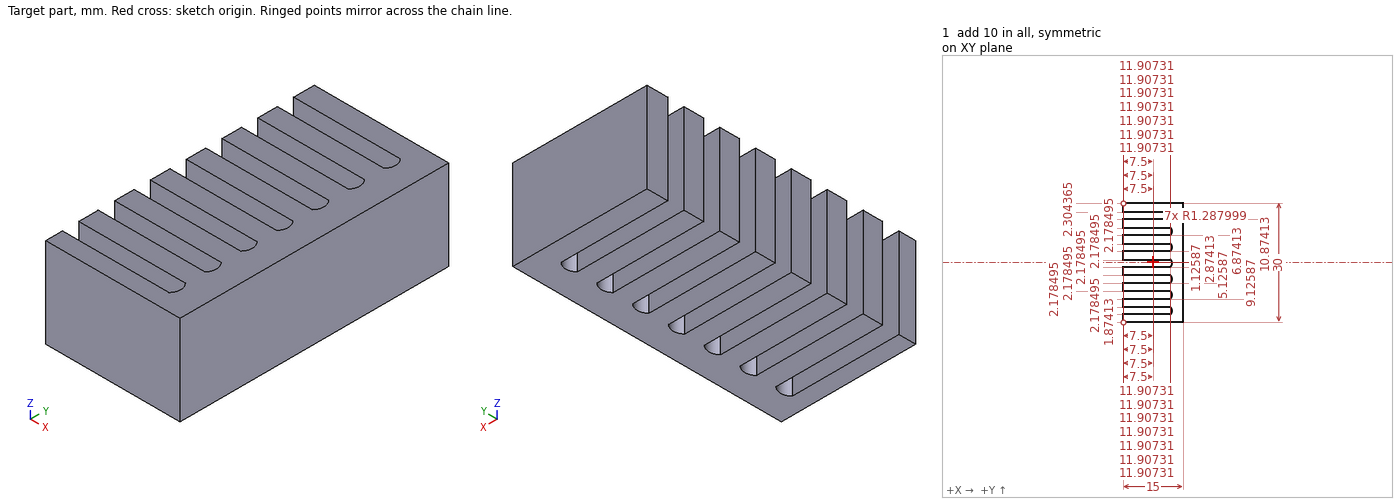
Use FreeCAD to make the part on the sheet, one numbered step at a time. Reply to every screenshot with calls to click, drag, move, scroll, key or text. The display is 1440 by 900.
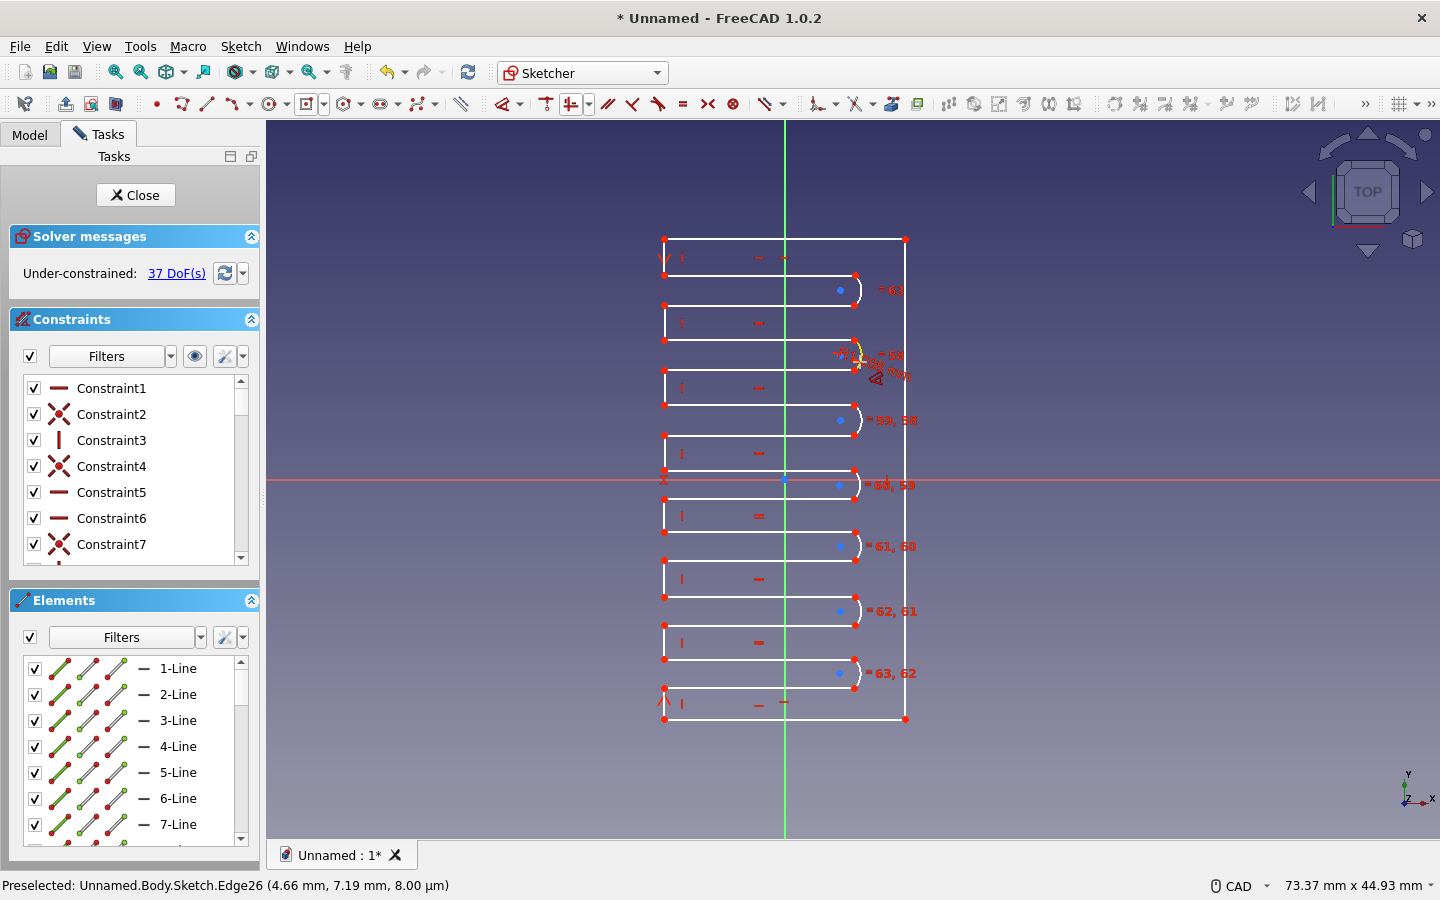
click(737, 720)
click(729, 754)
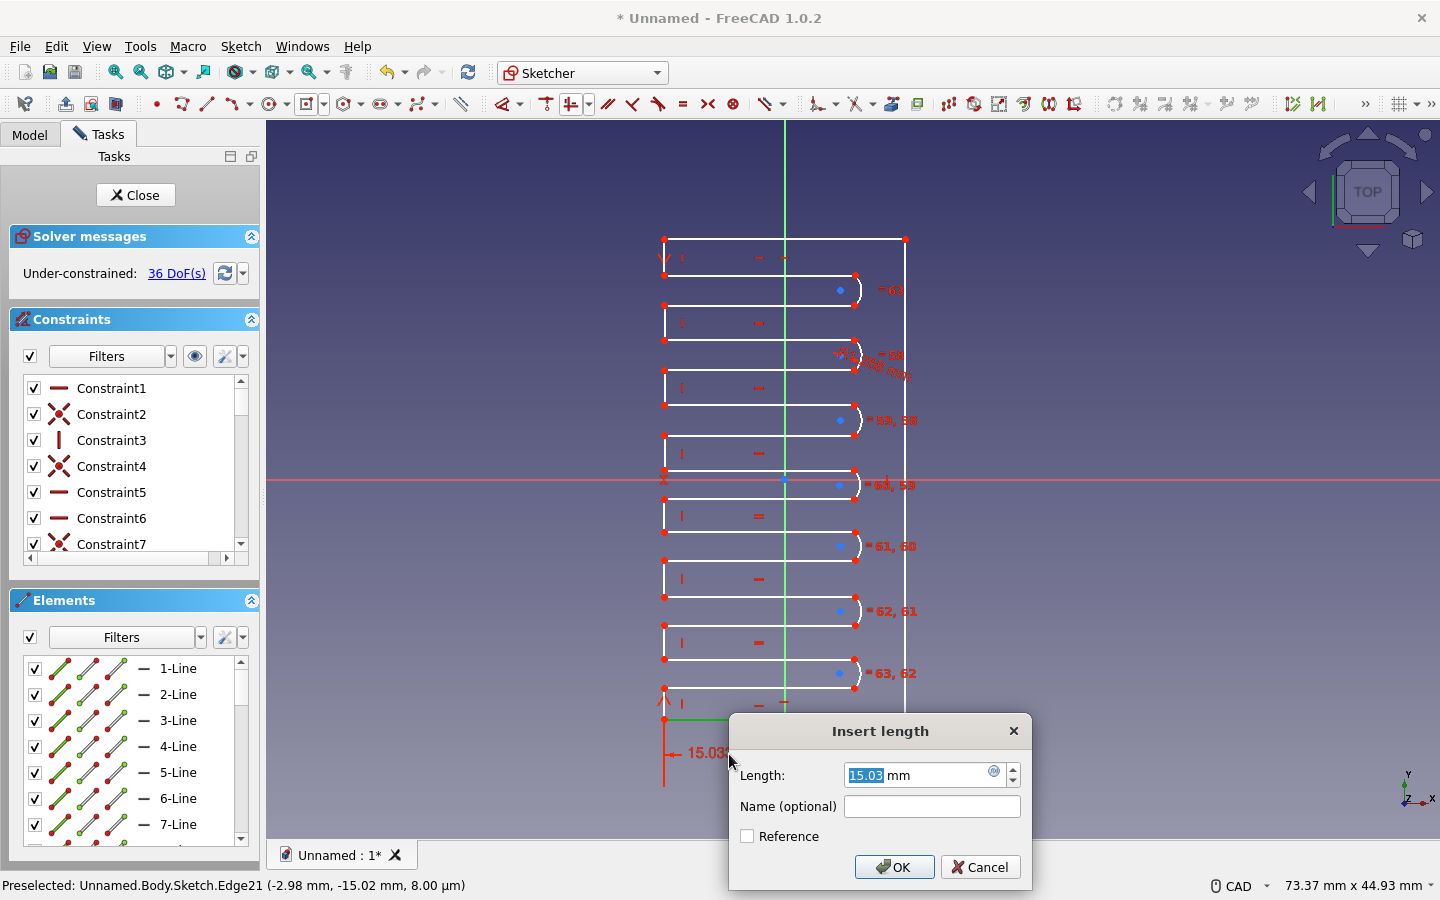
text(15)
key(Return)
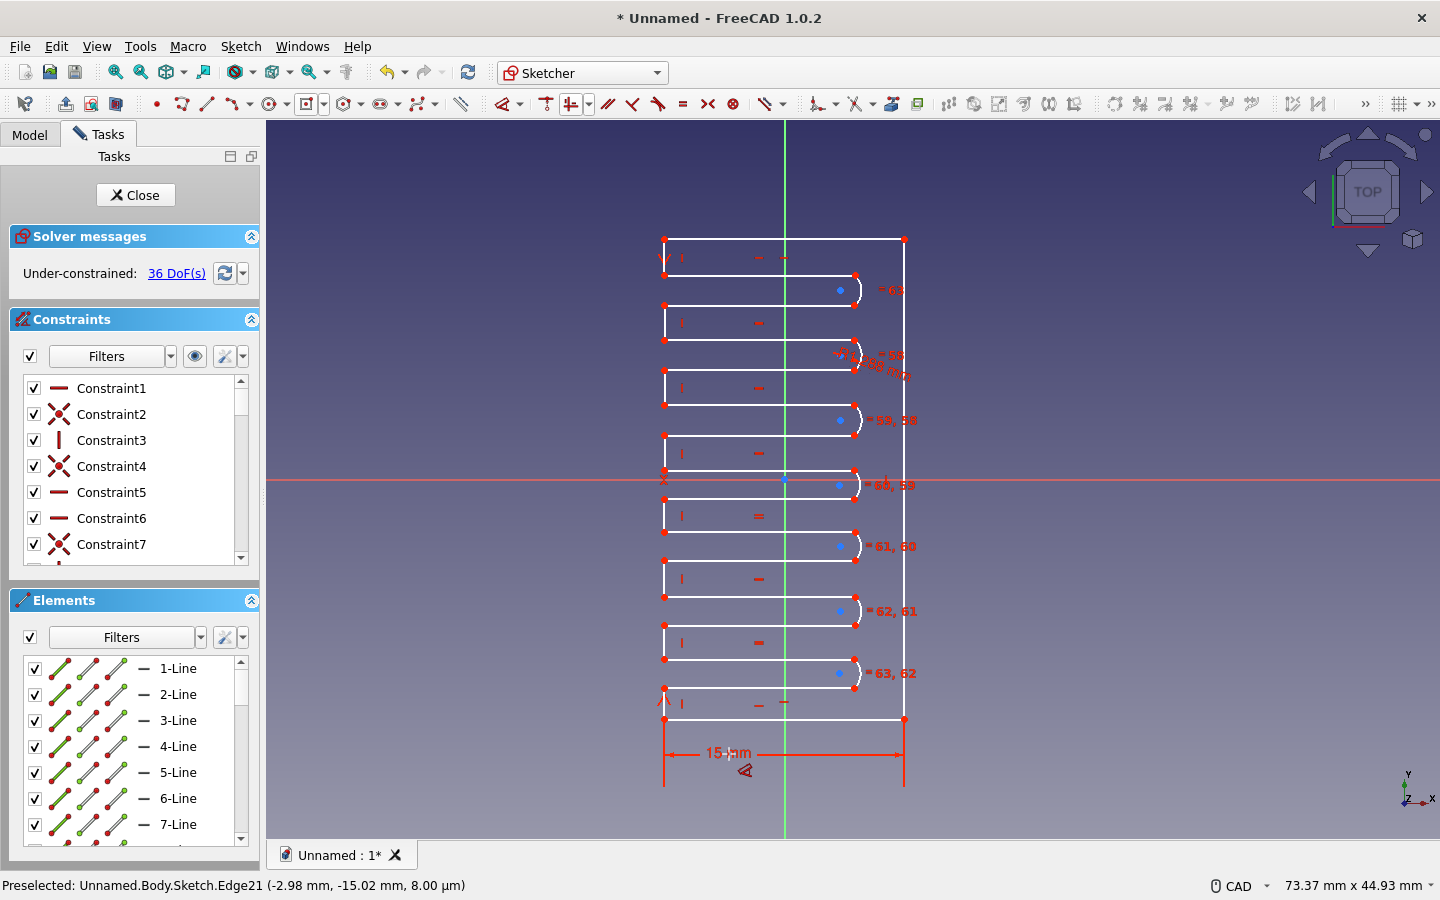
click(904, 576)
click(938, 590)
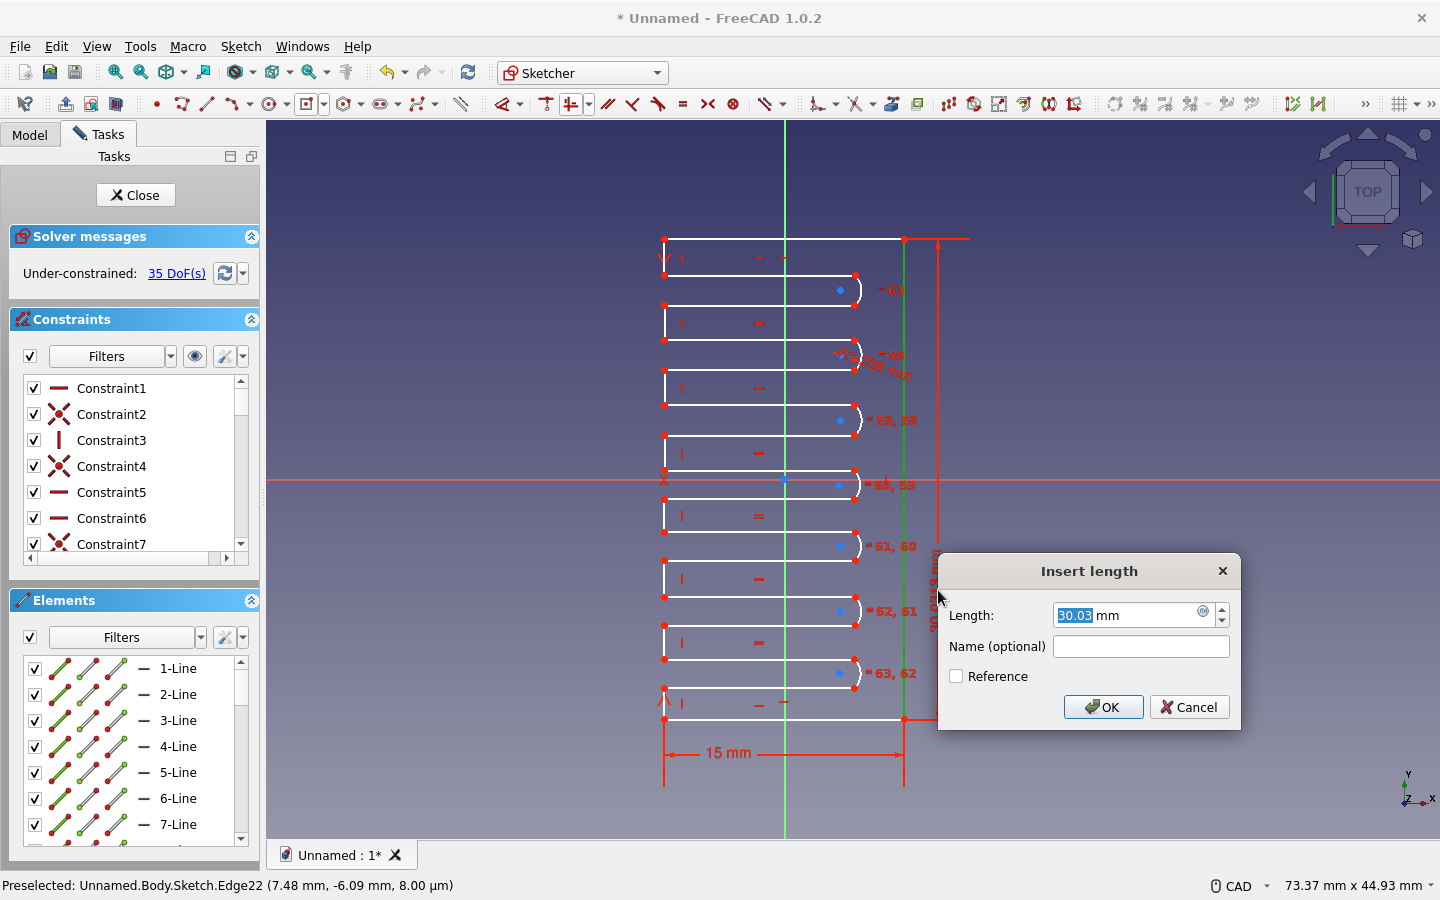
text(30)
key(Return)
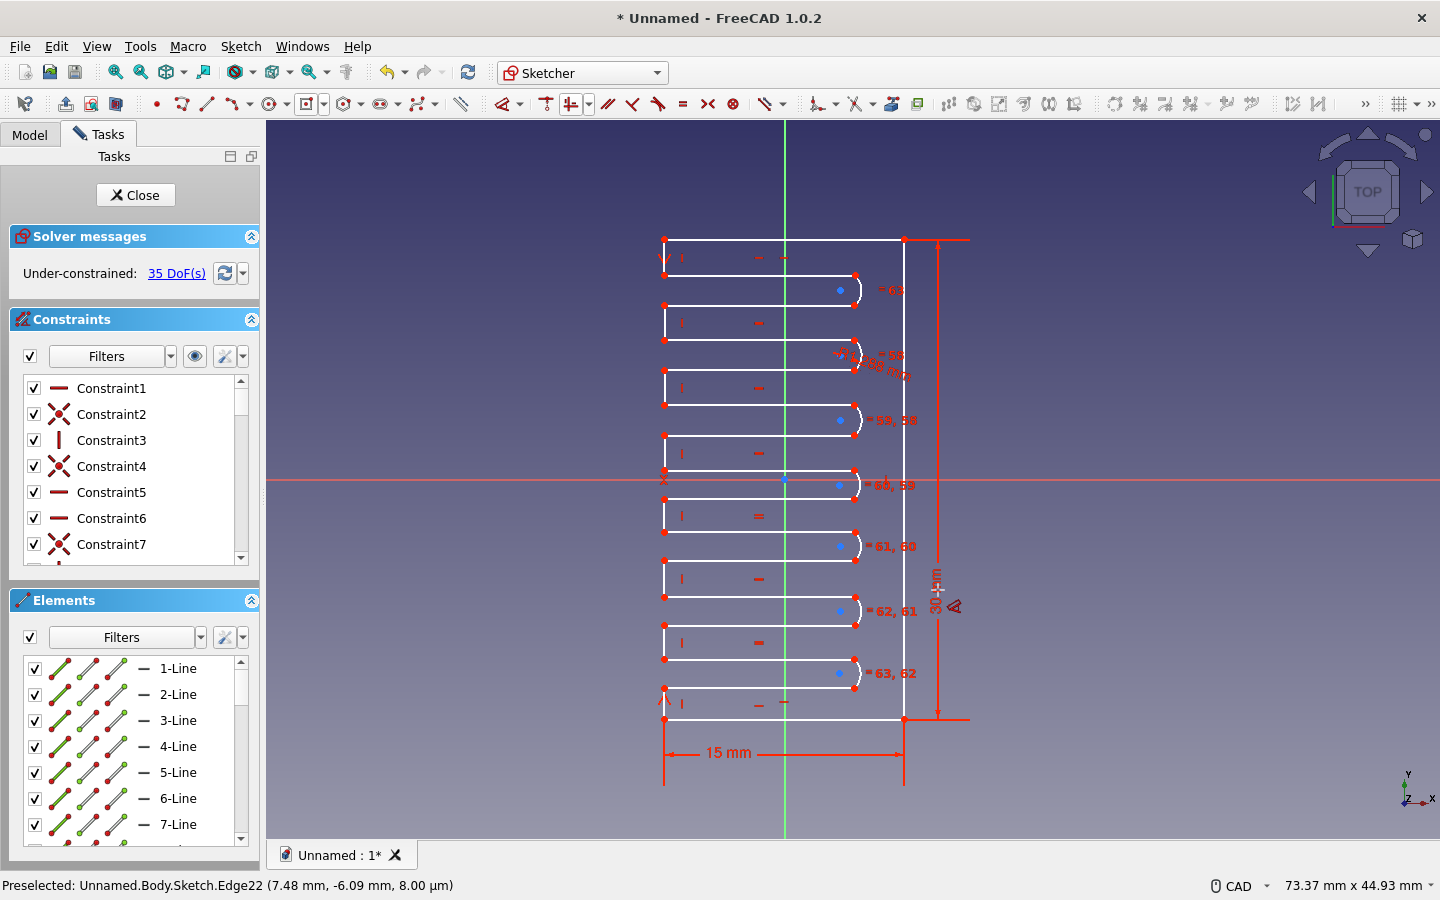
click(665, 306)
click(725, 514)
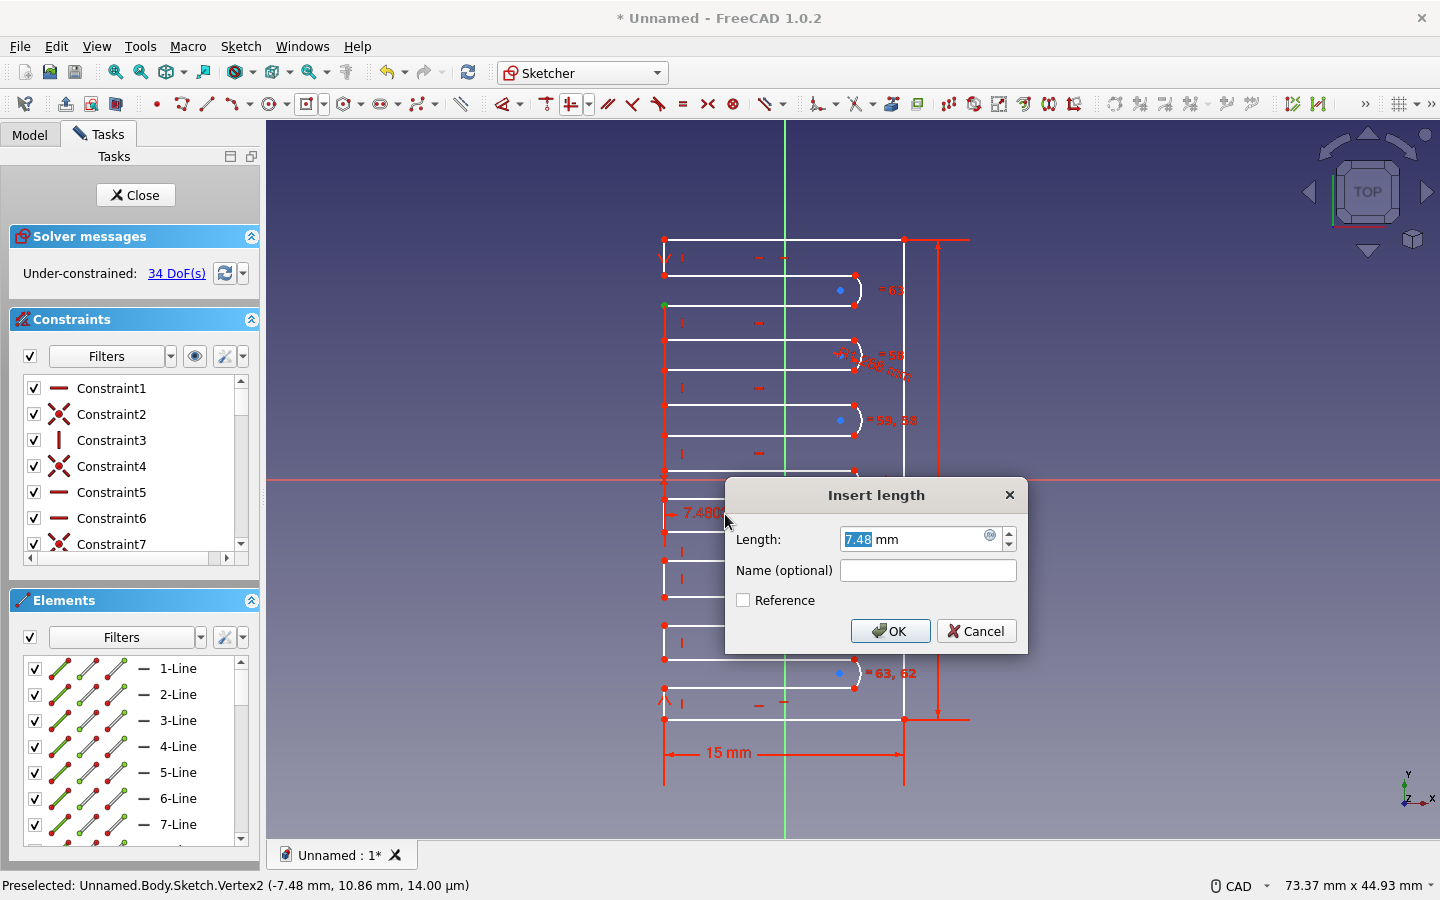
text(7.5)
key(Return)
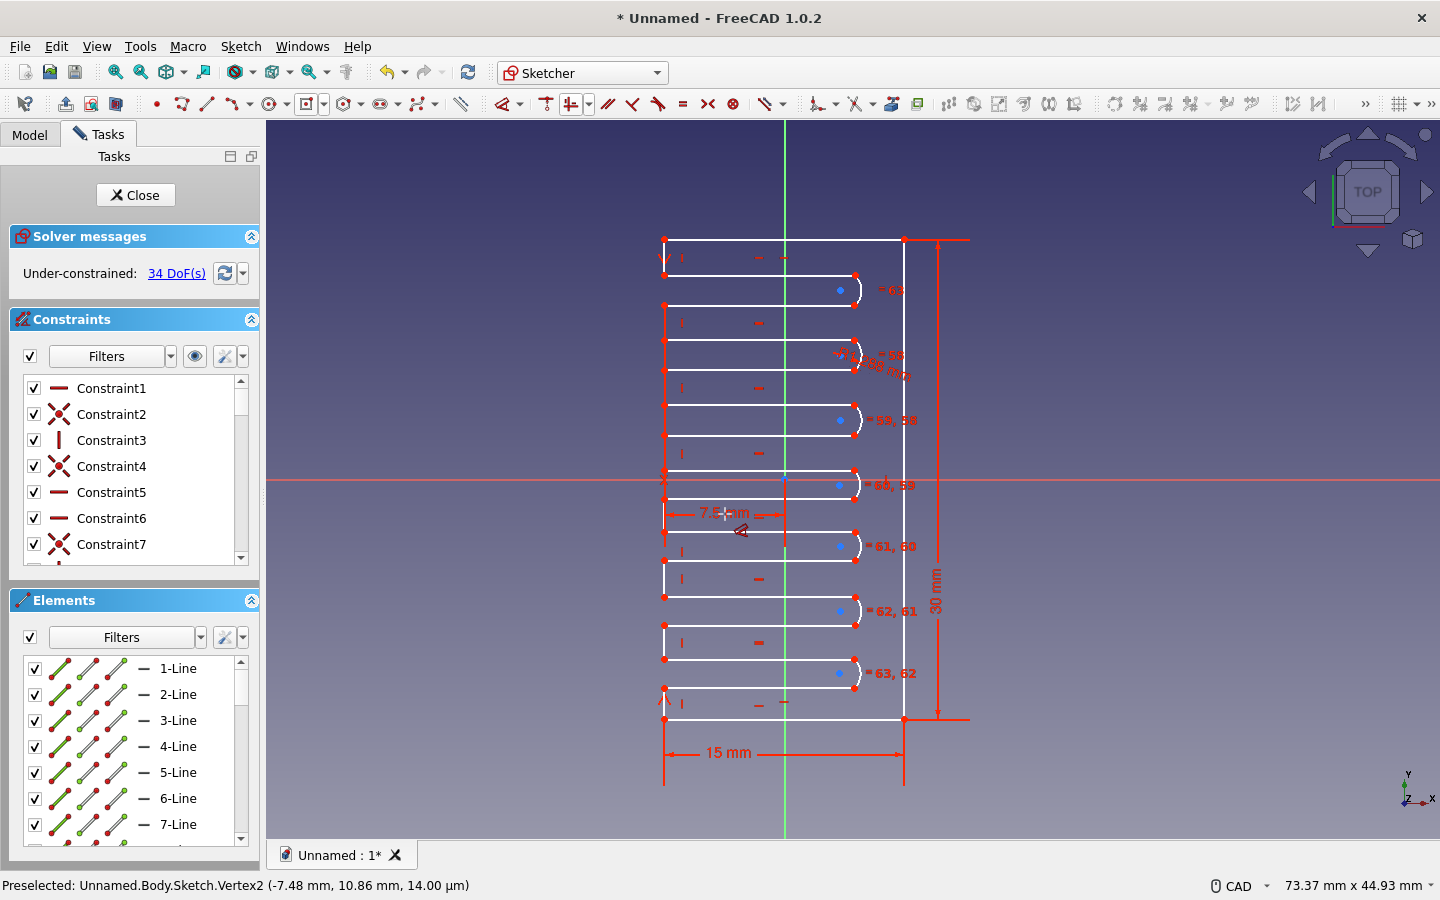
click(665, 370)
click(725, 216)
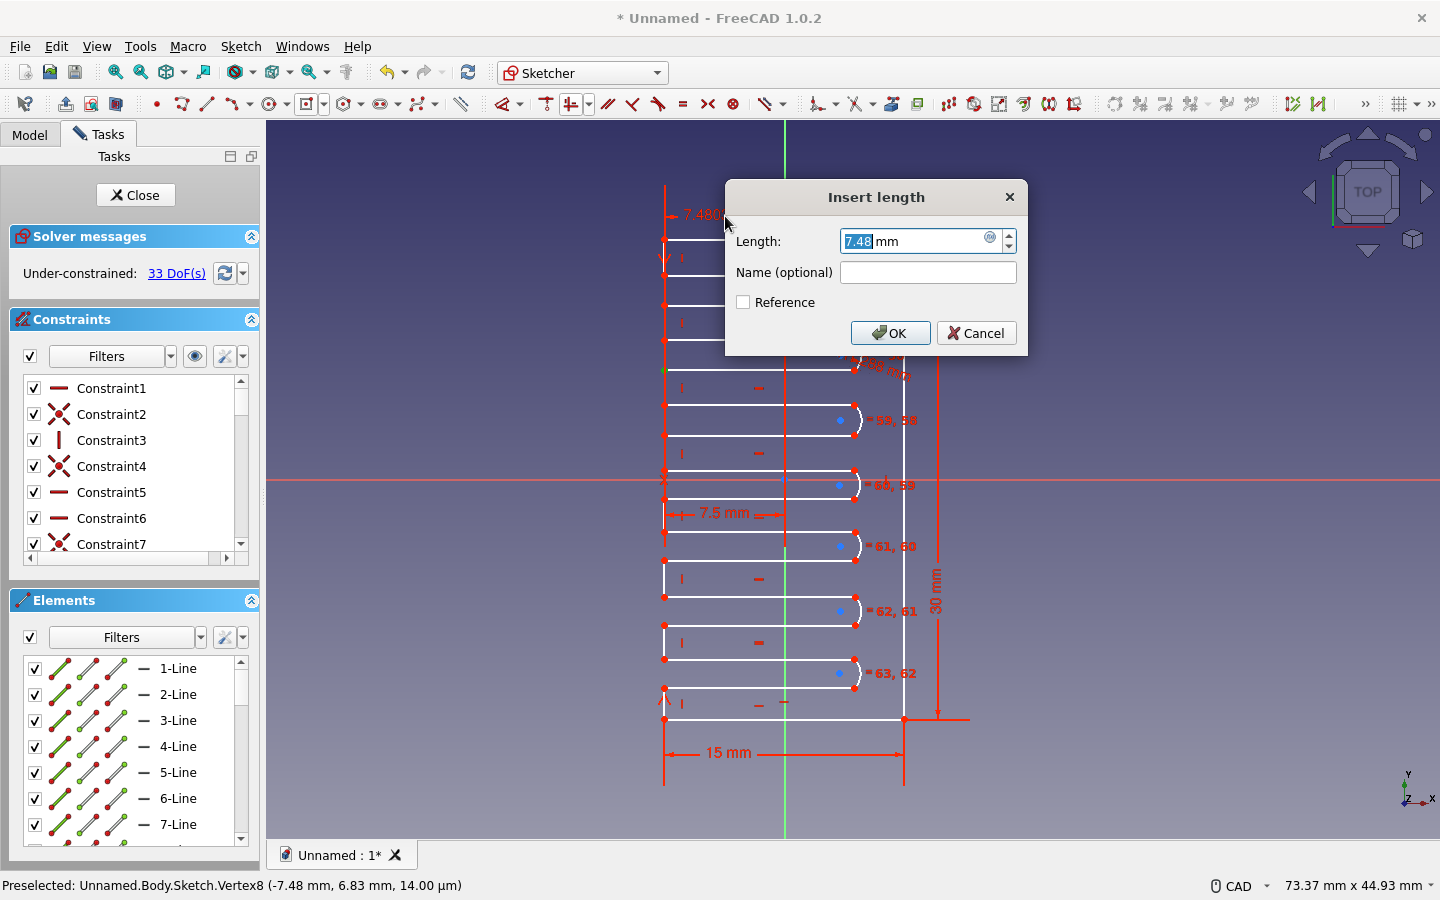
text(7.5)
key(Return)